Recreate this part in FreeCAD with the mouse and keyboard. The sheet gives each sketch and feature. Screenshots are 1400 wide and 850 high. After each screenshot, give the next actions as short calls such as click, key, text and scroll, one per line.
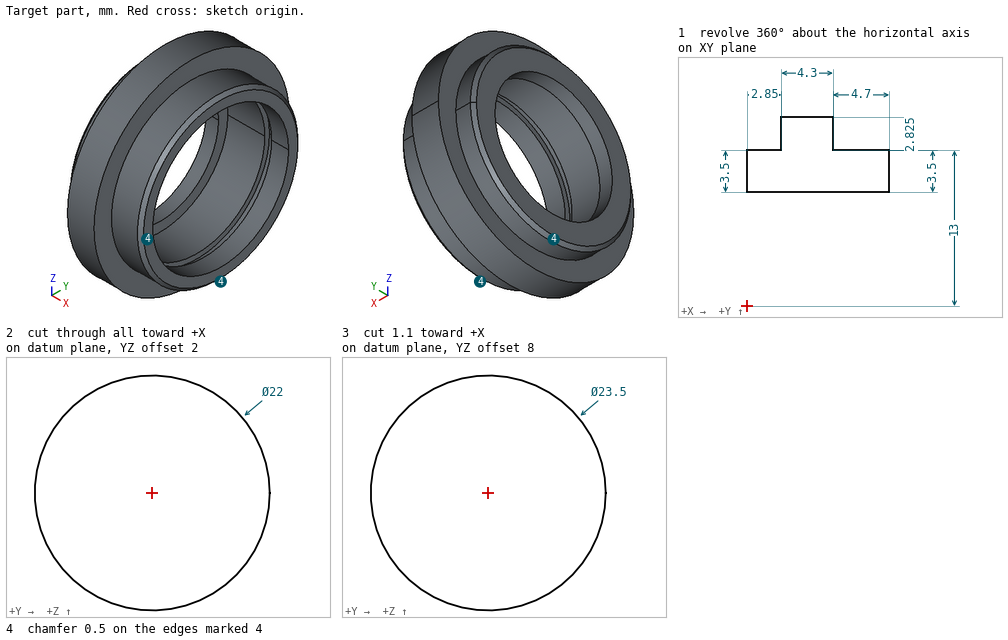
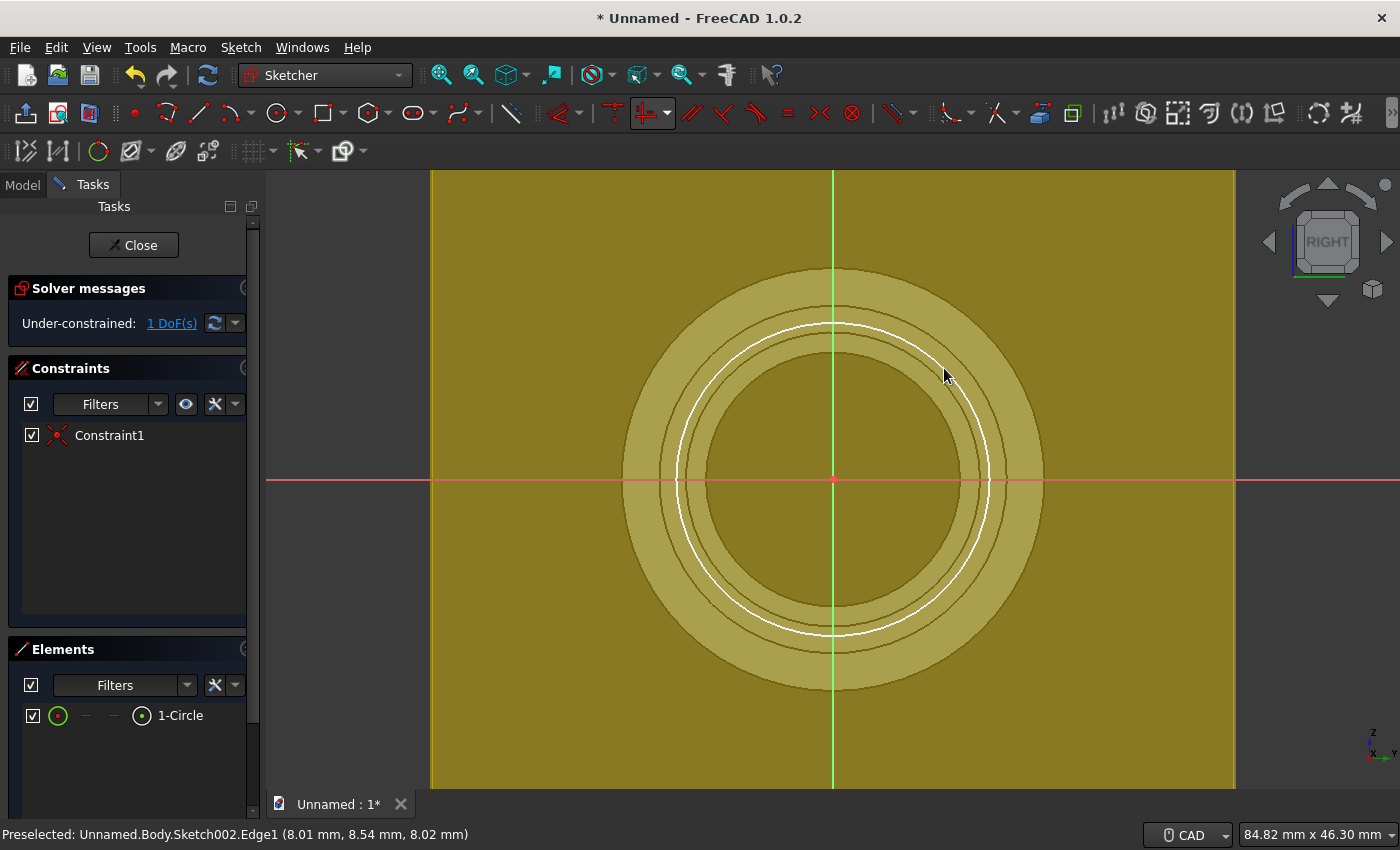
click(558, 114)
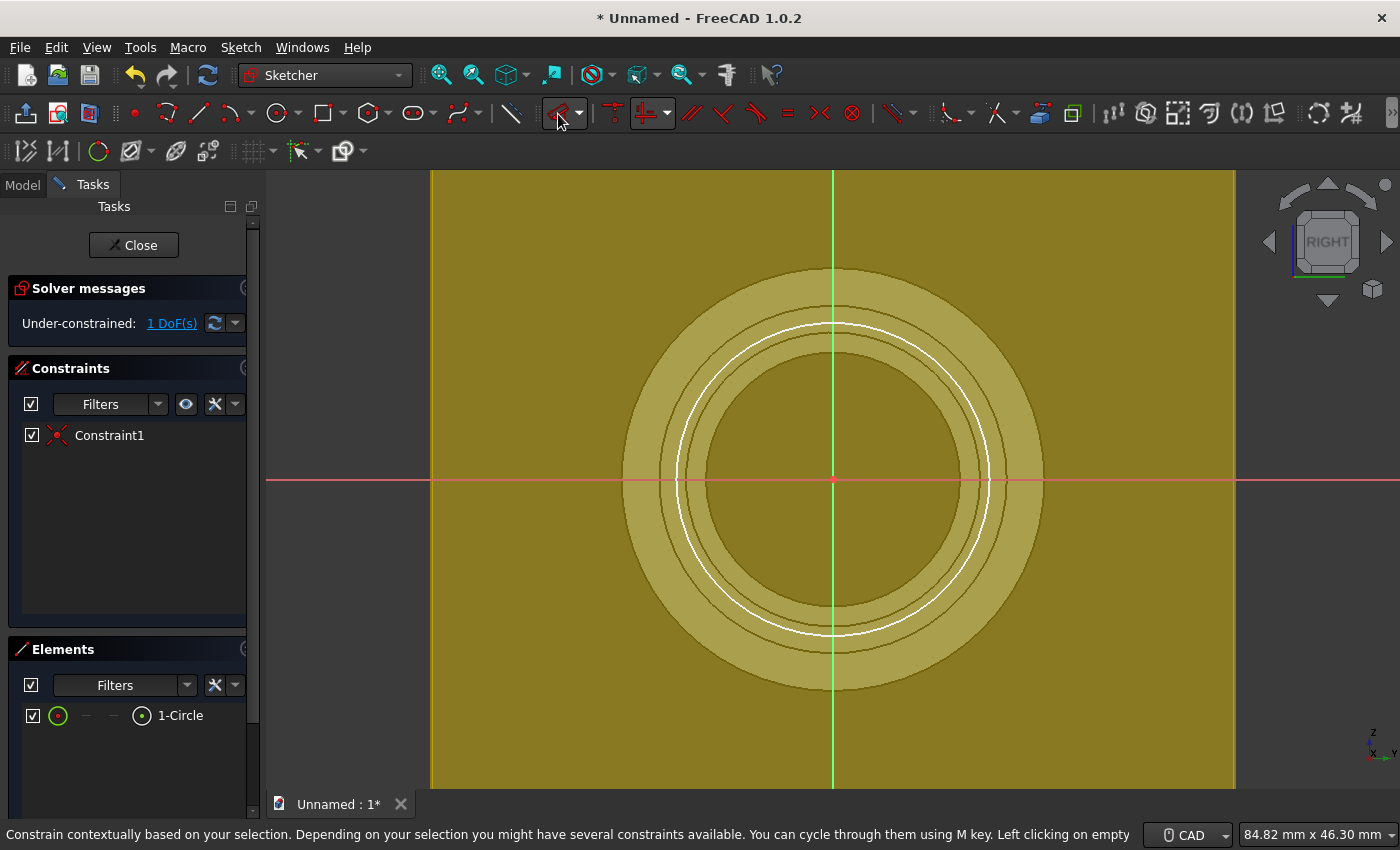
click(943, 368)
click(965, 345)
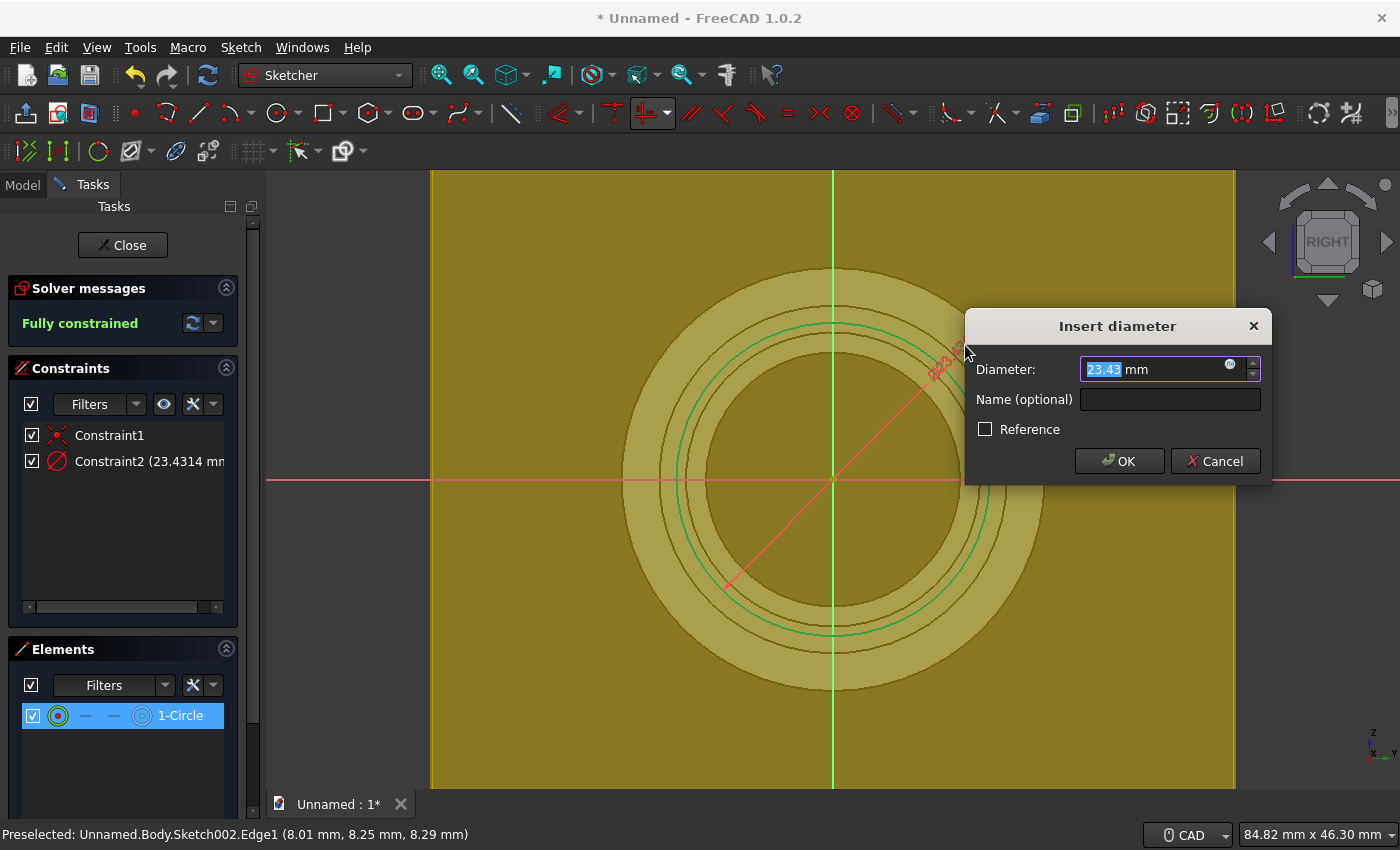
text(23.5)
key(Return)
key(Escape)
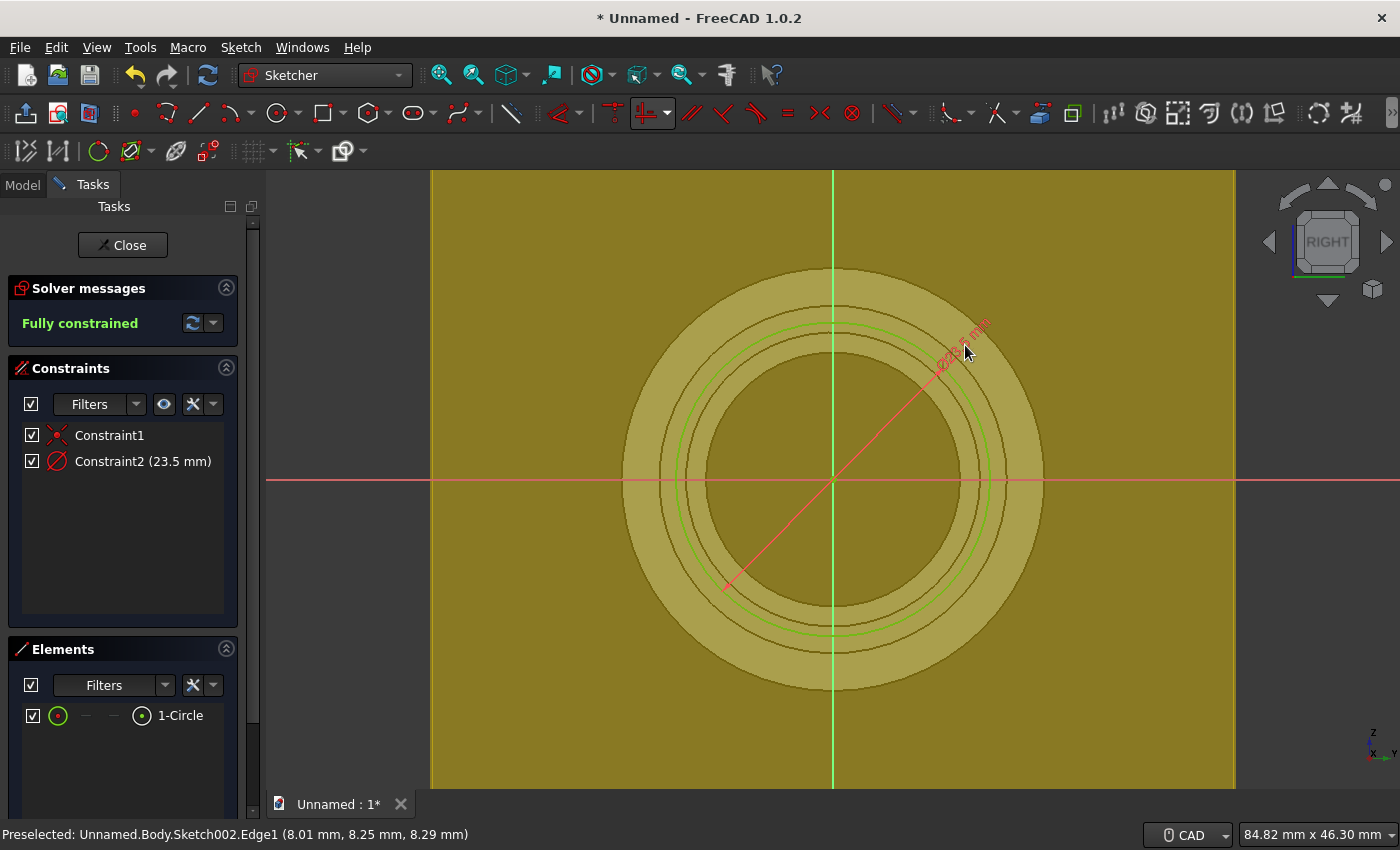
click(123, 245)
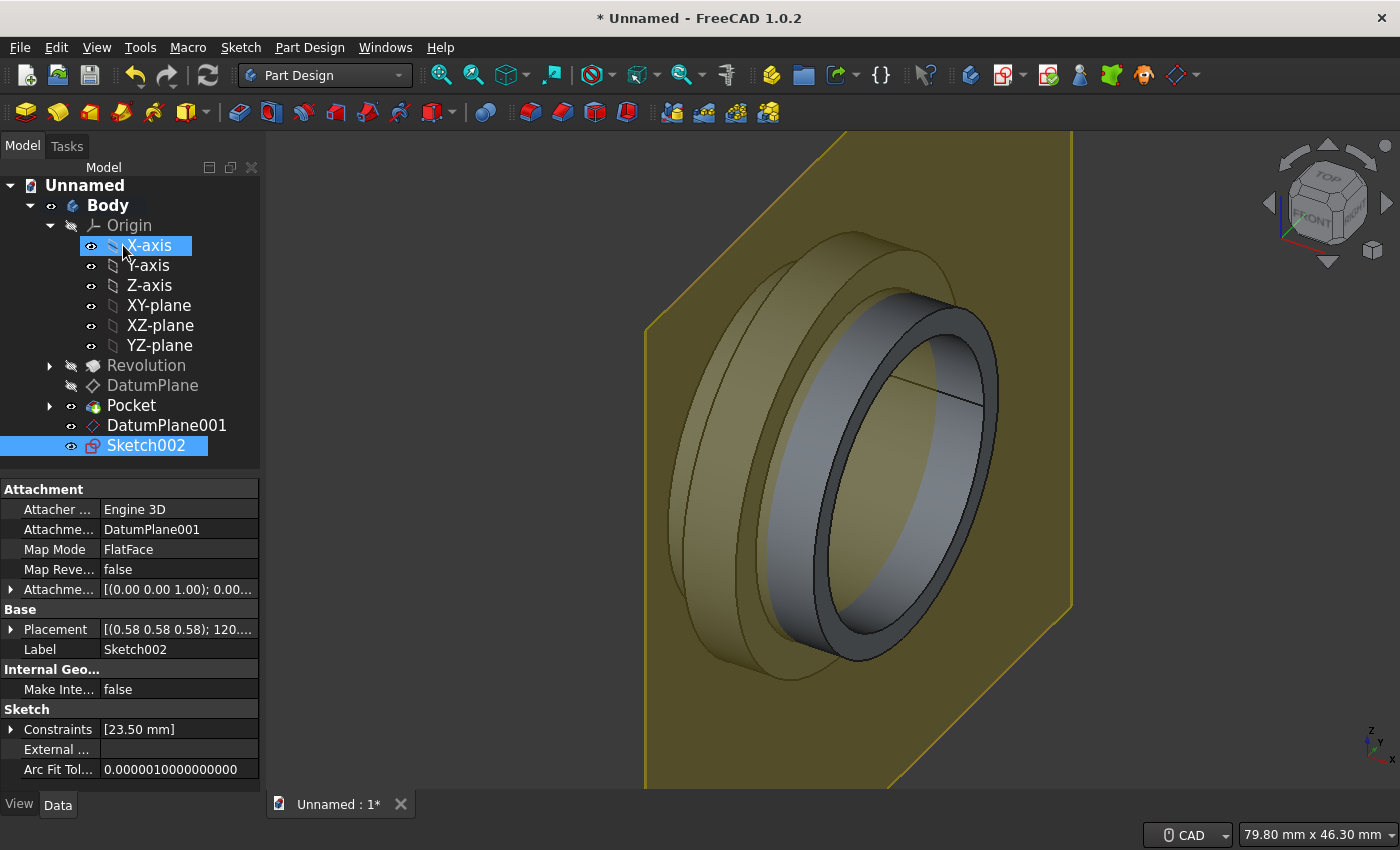
click(240, 112)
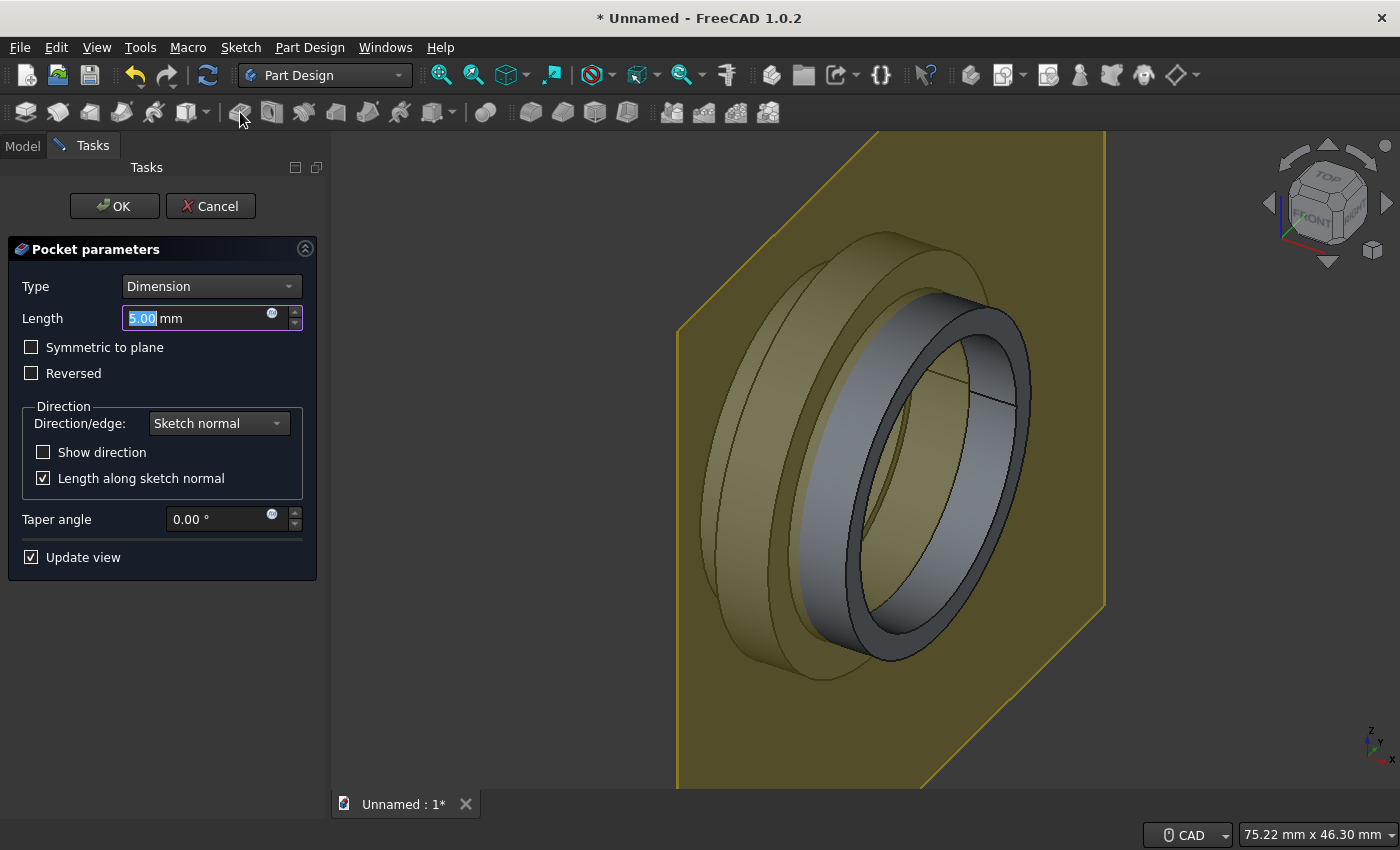
text(1.1)
key(Tab)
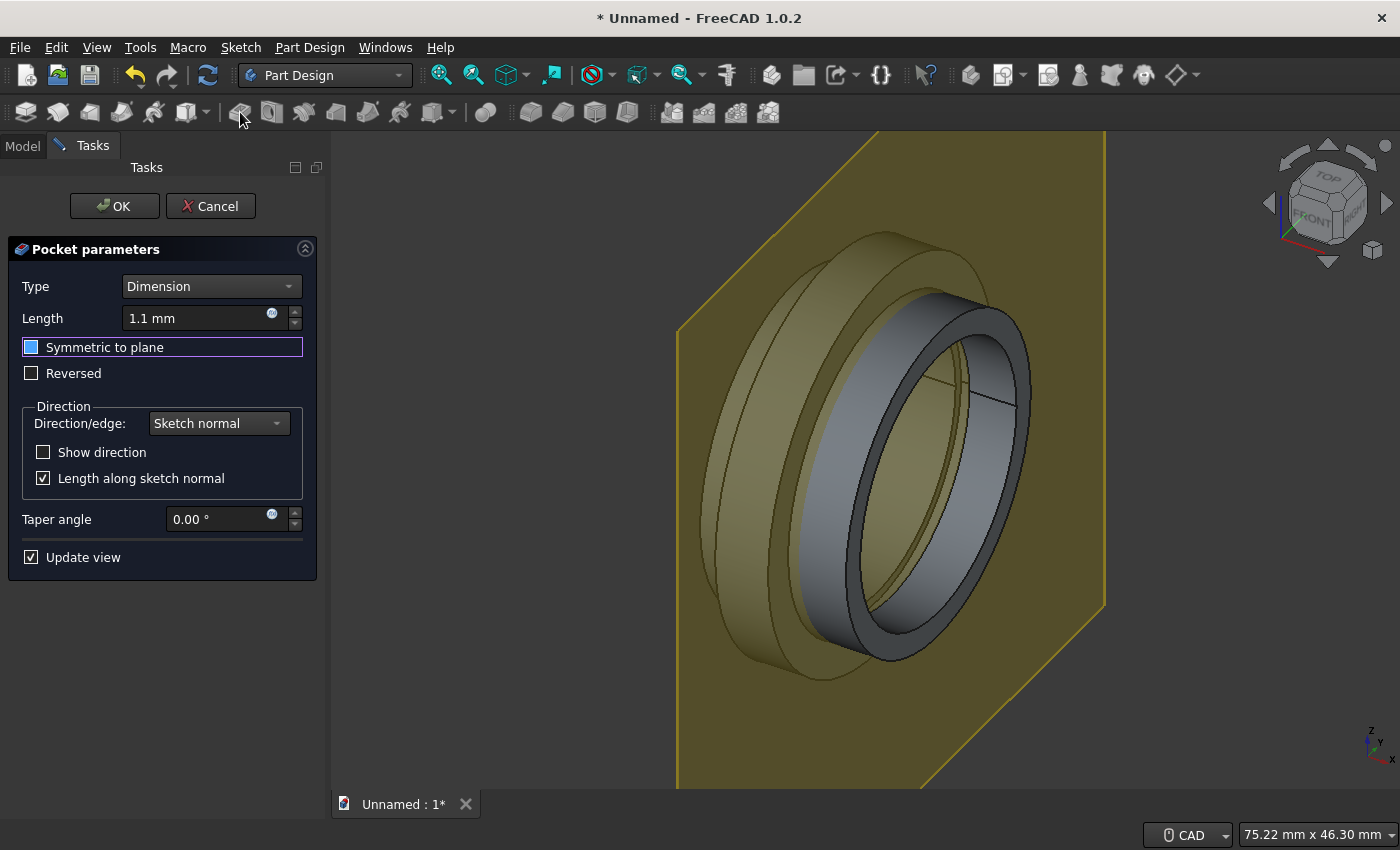
click(30, 373)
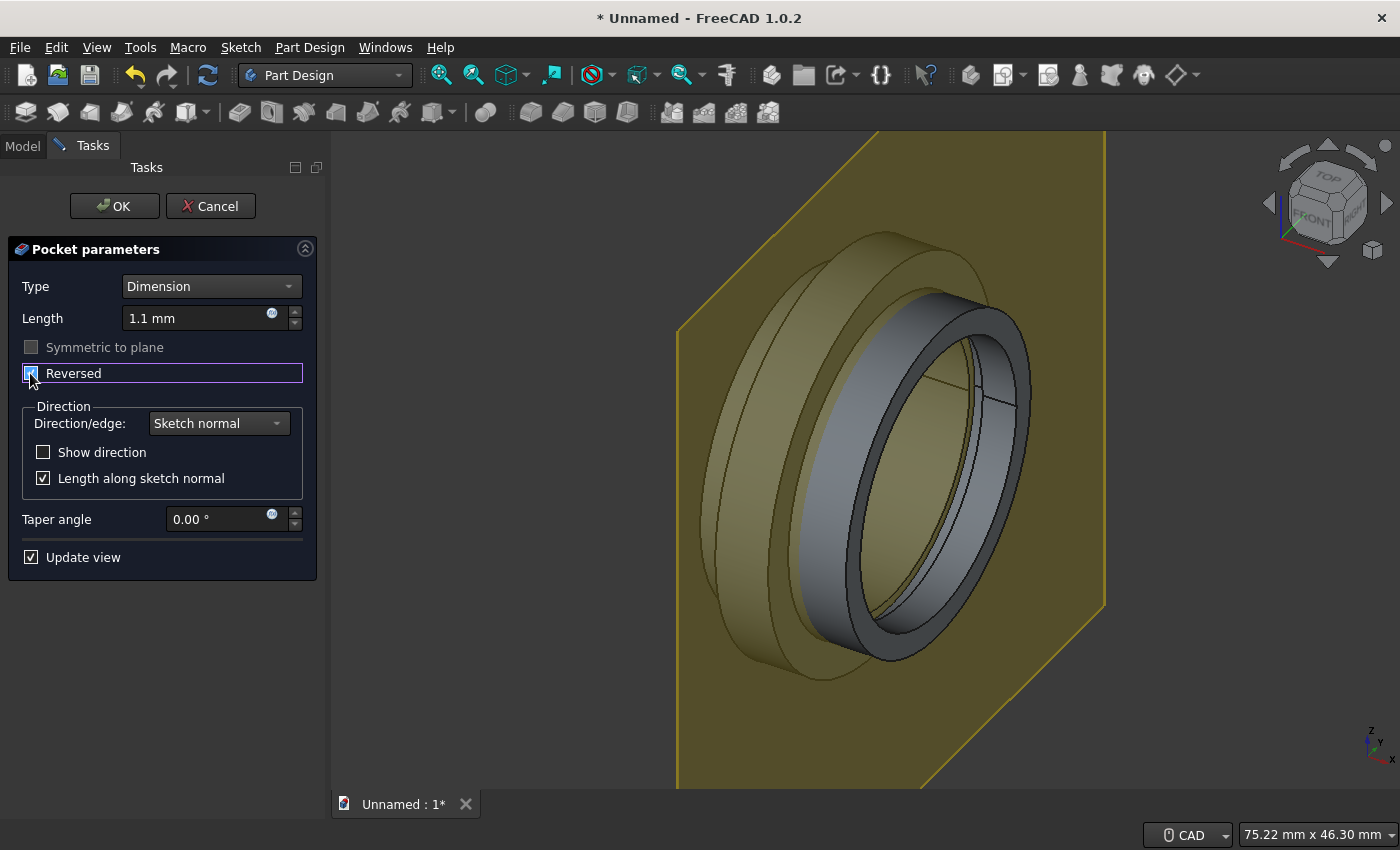
click(115, 206)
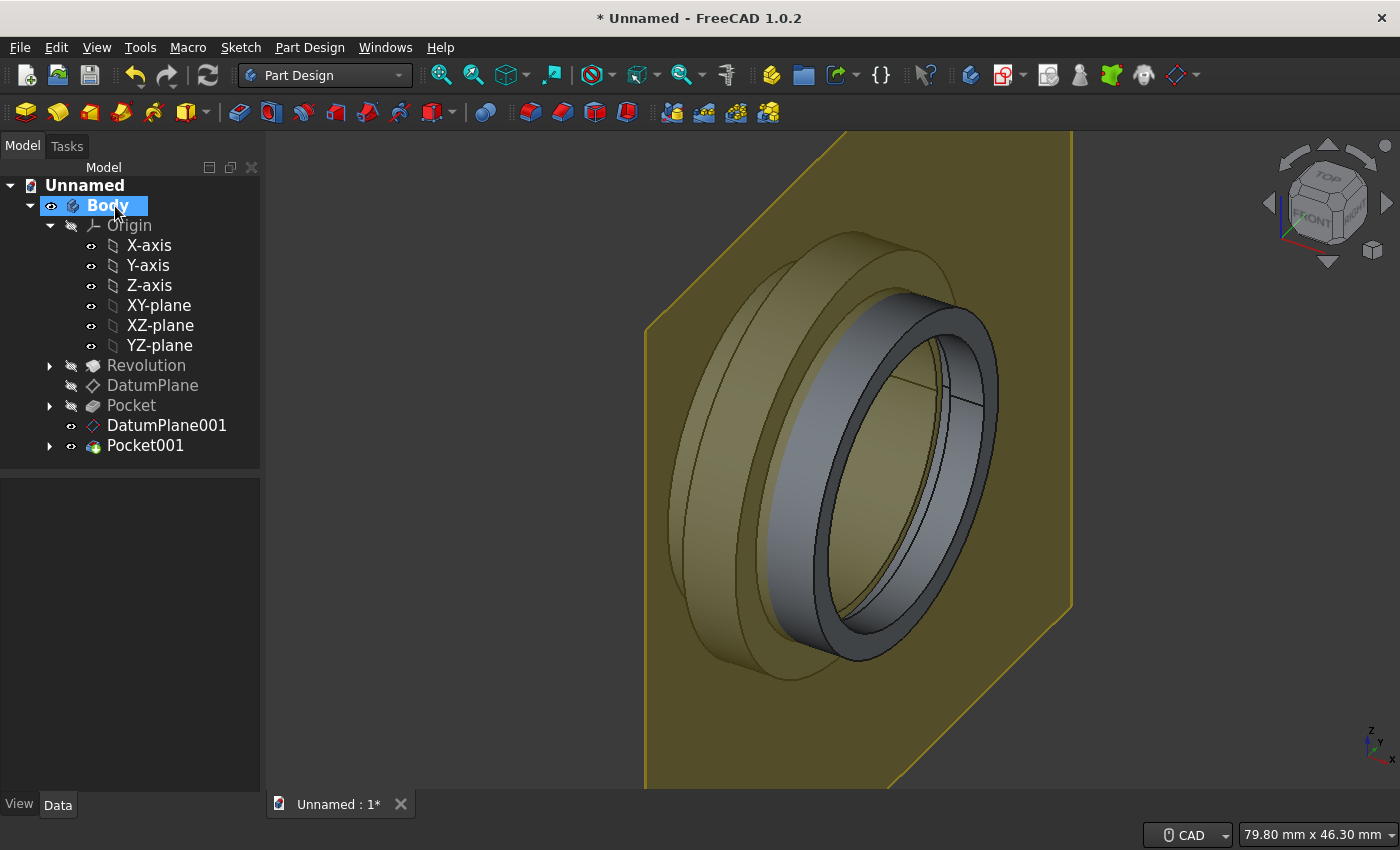
click(116, 426)
key(space)